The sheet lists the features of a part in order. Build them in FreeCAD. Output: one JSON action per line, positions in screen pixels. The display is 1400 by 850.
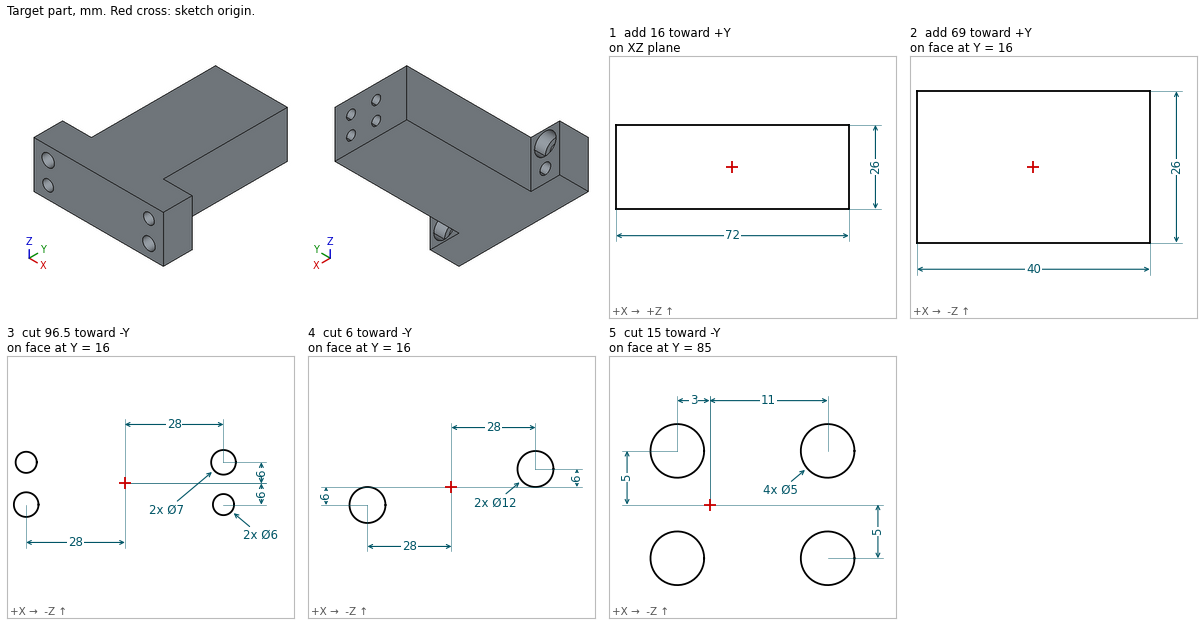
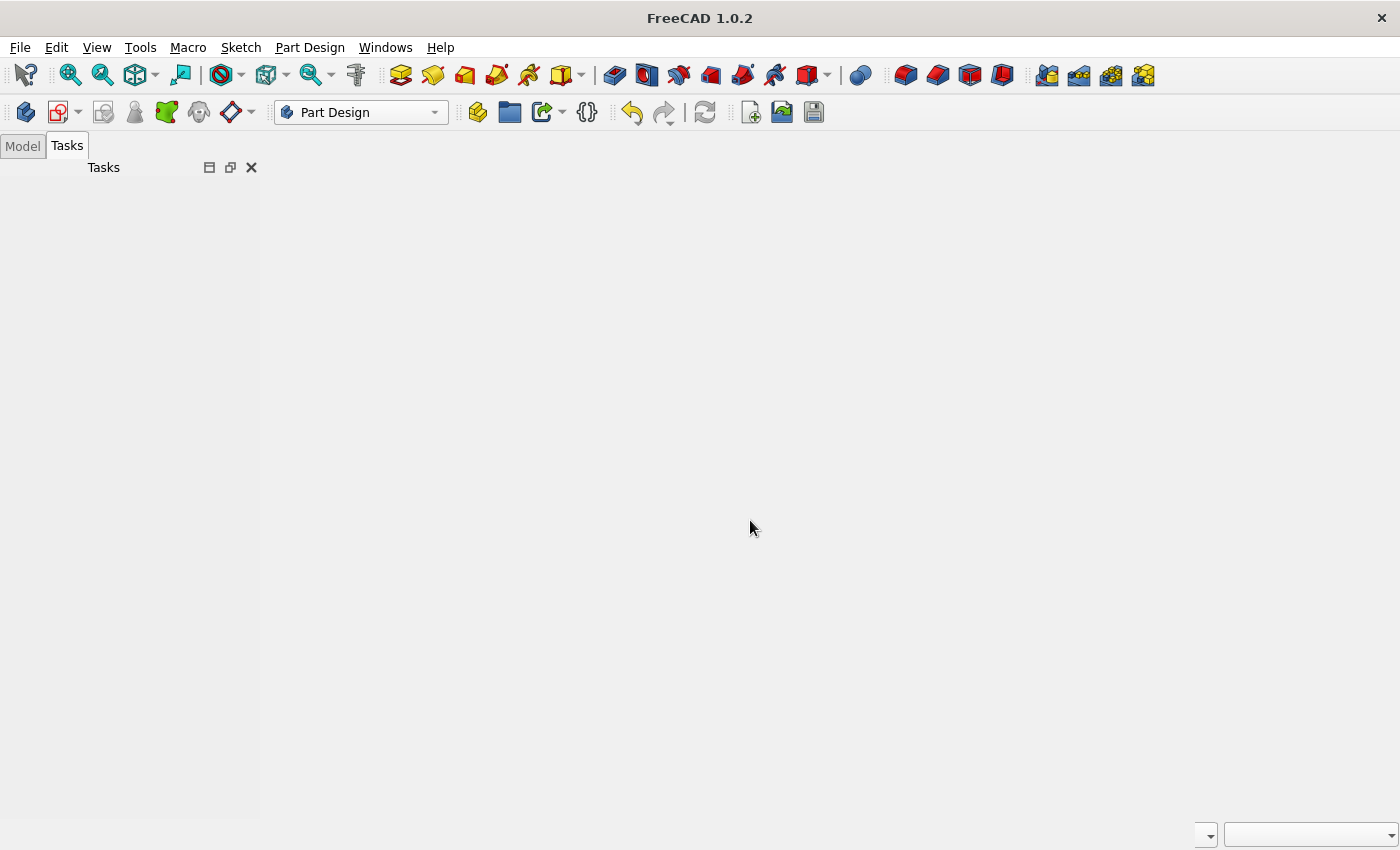
{"action": "left_click", "coordinate": [750, 112]}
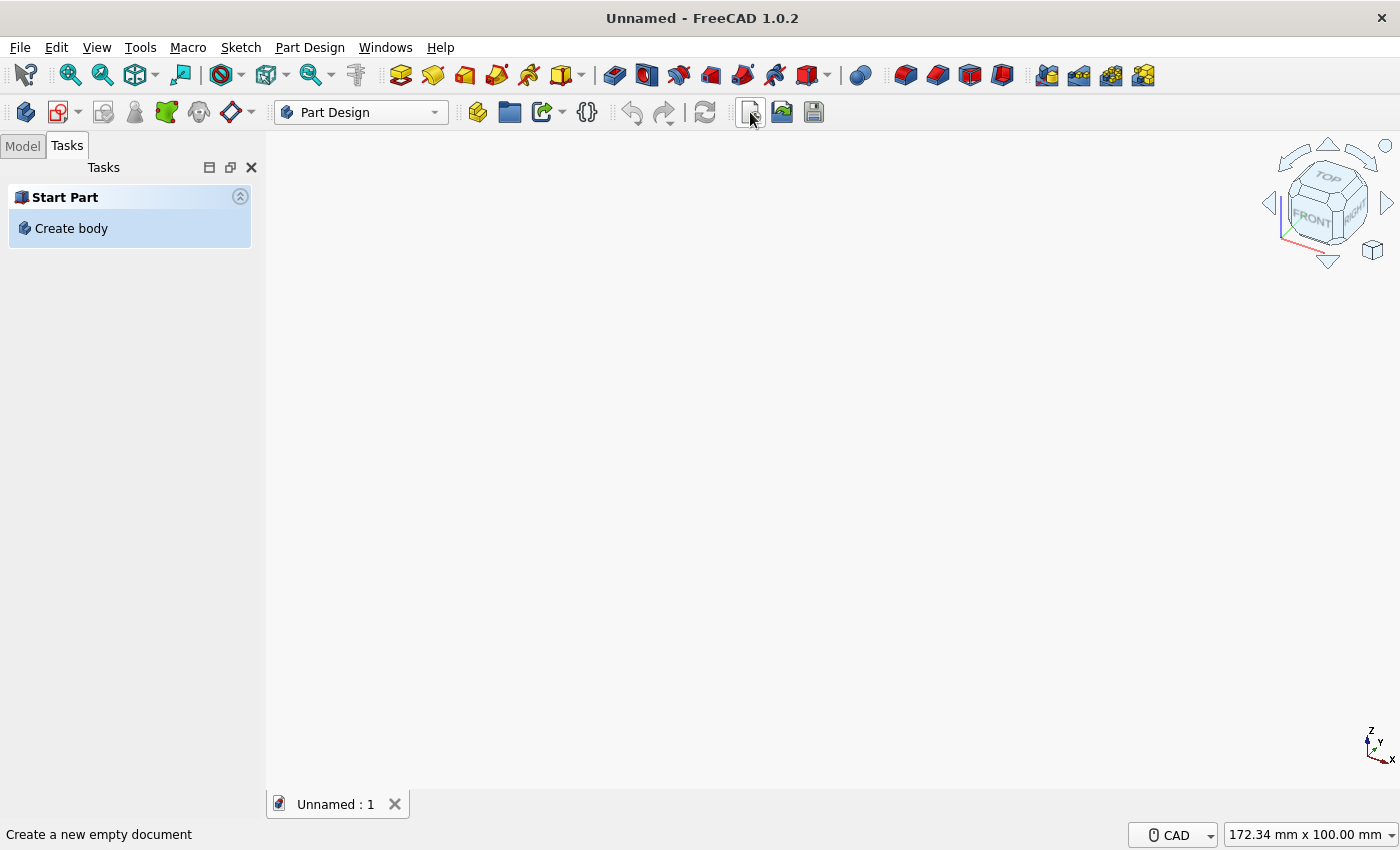
{"action": "left_click", "coordinate": [58, 112]}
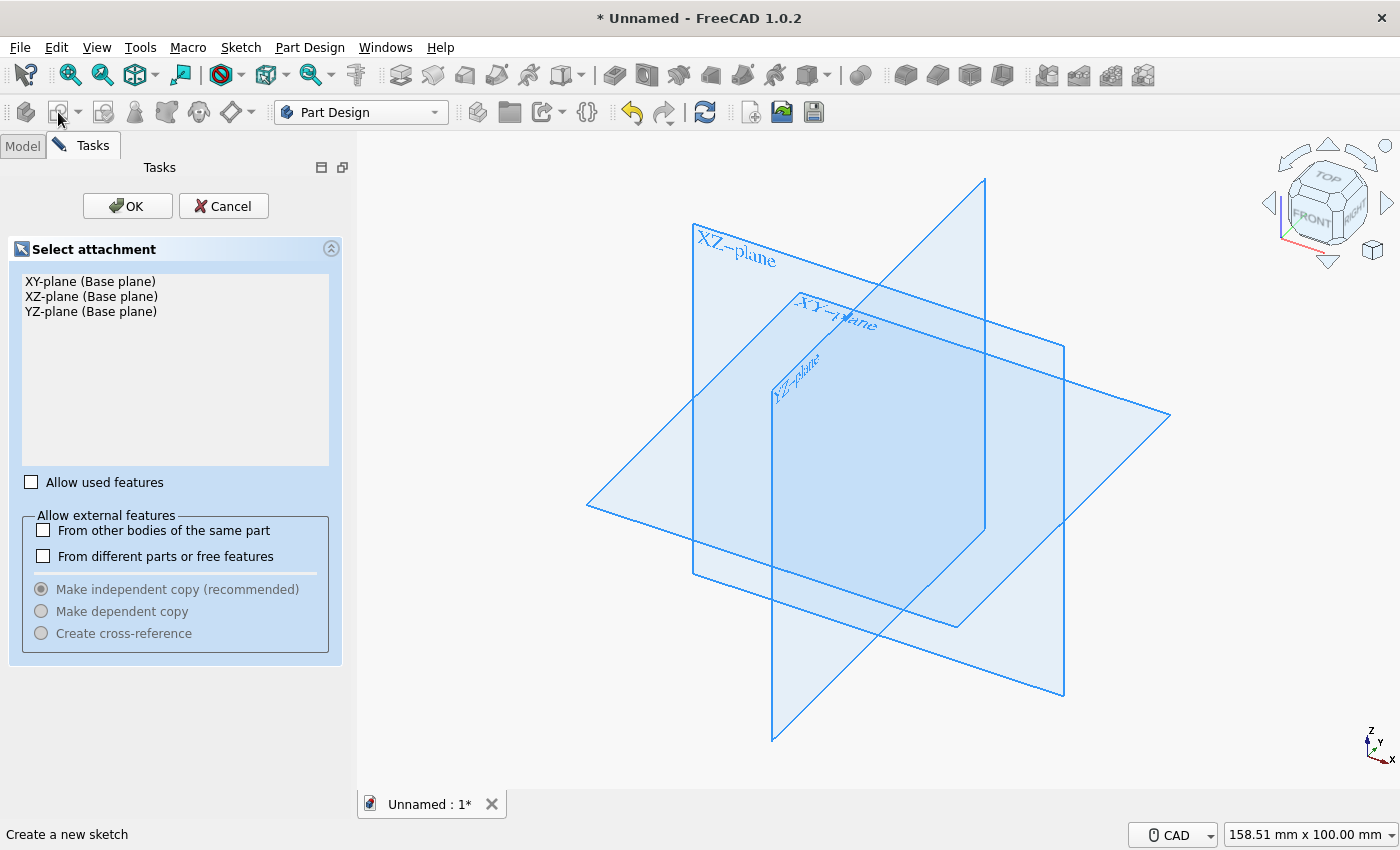
{"action": "left_click", "coordinate": [82, 296]}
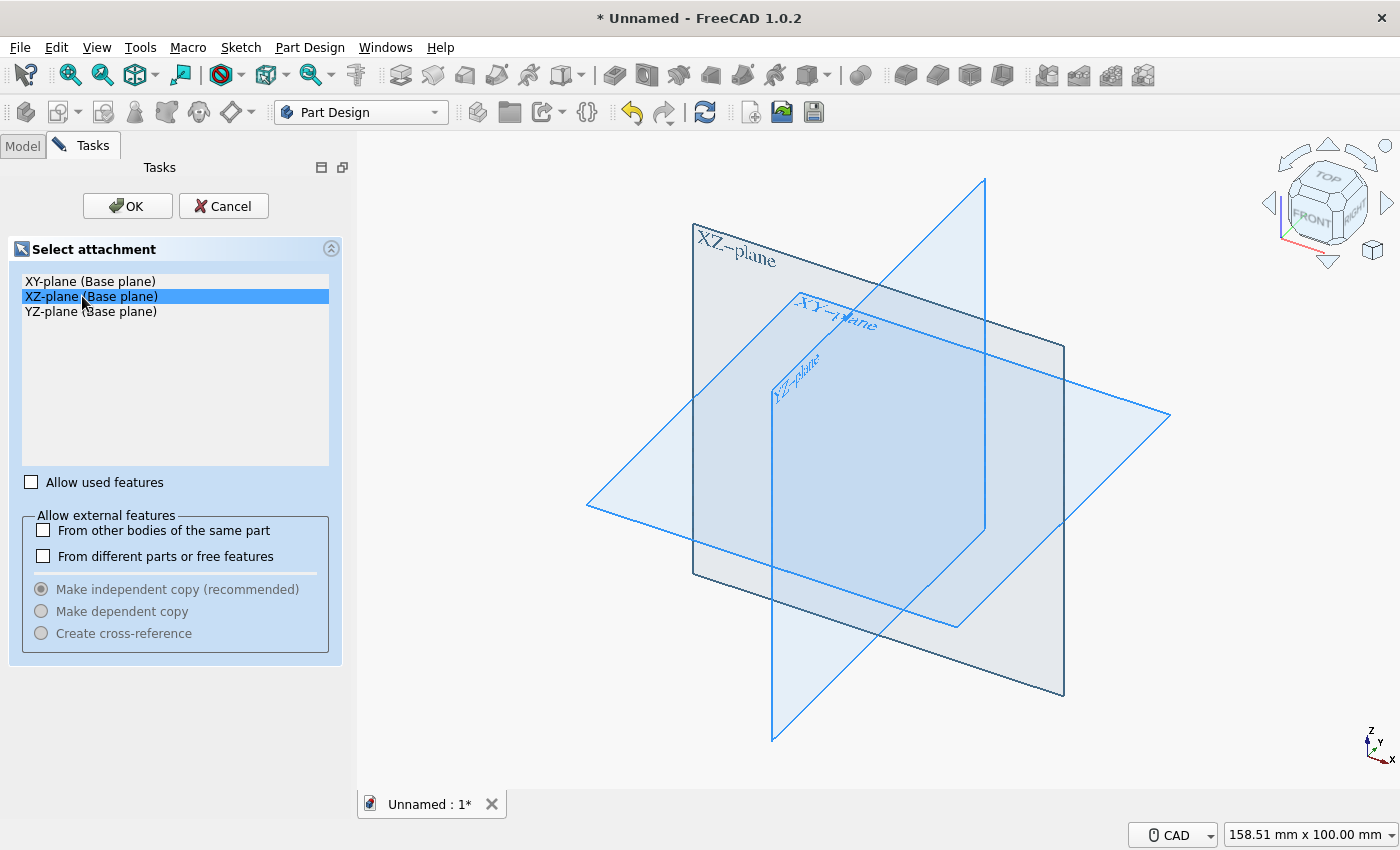
{"action": "left_click", "coordinate": [128, 206]}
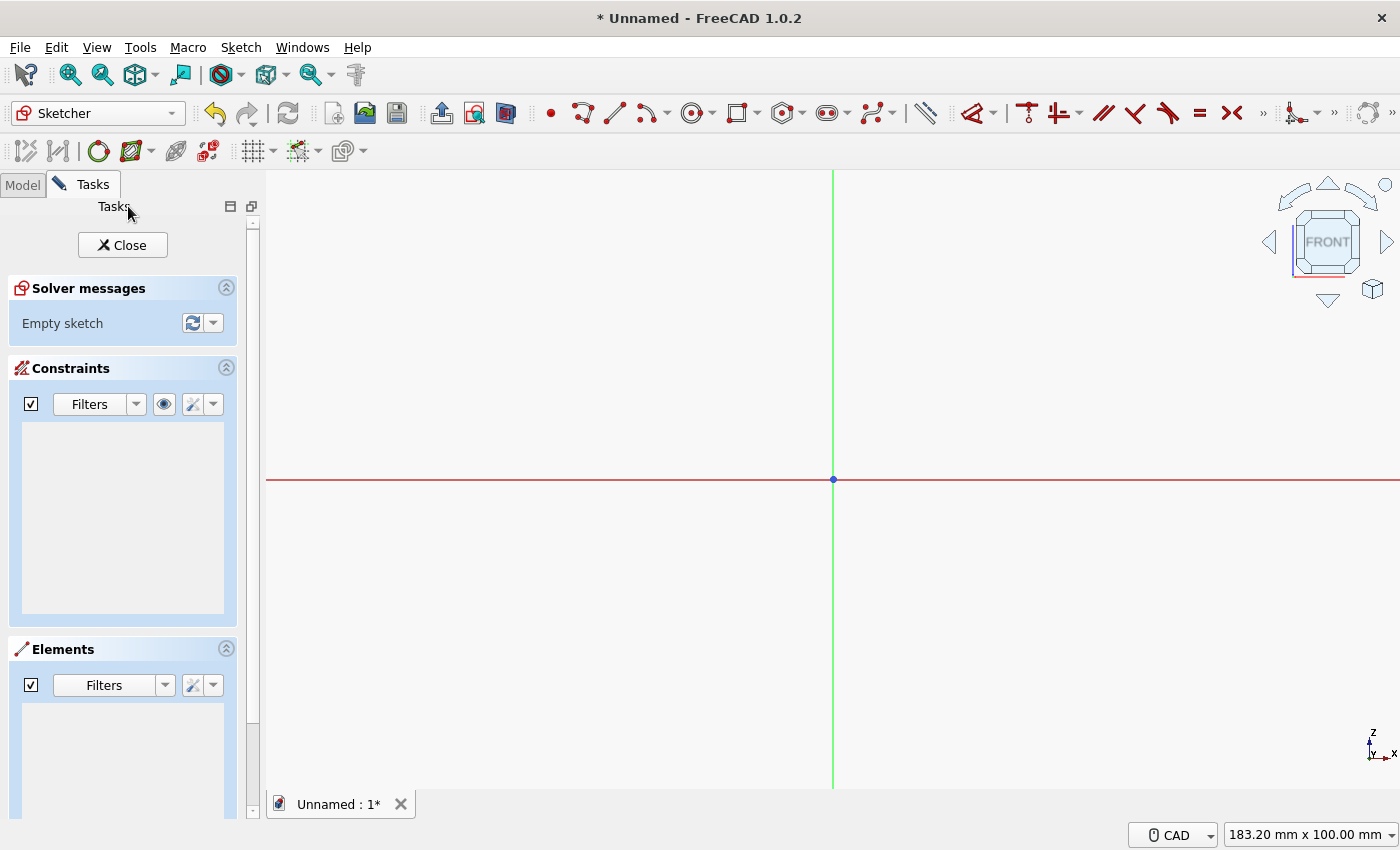
{"action": "scroll", "coordinate": [972, 480], "scroll_direction": "up", "scroll_amount": 2}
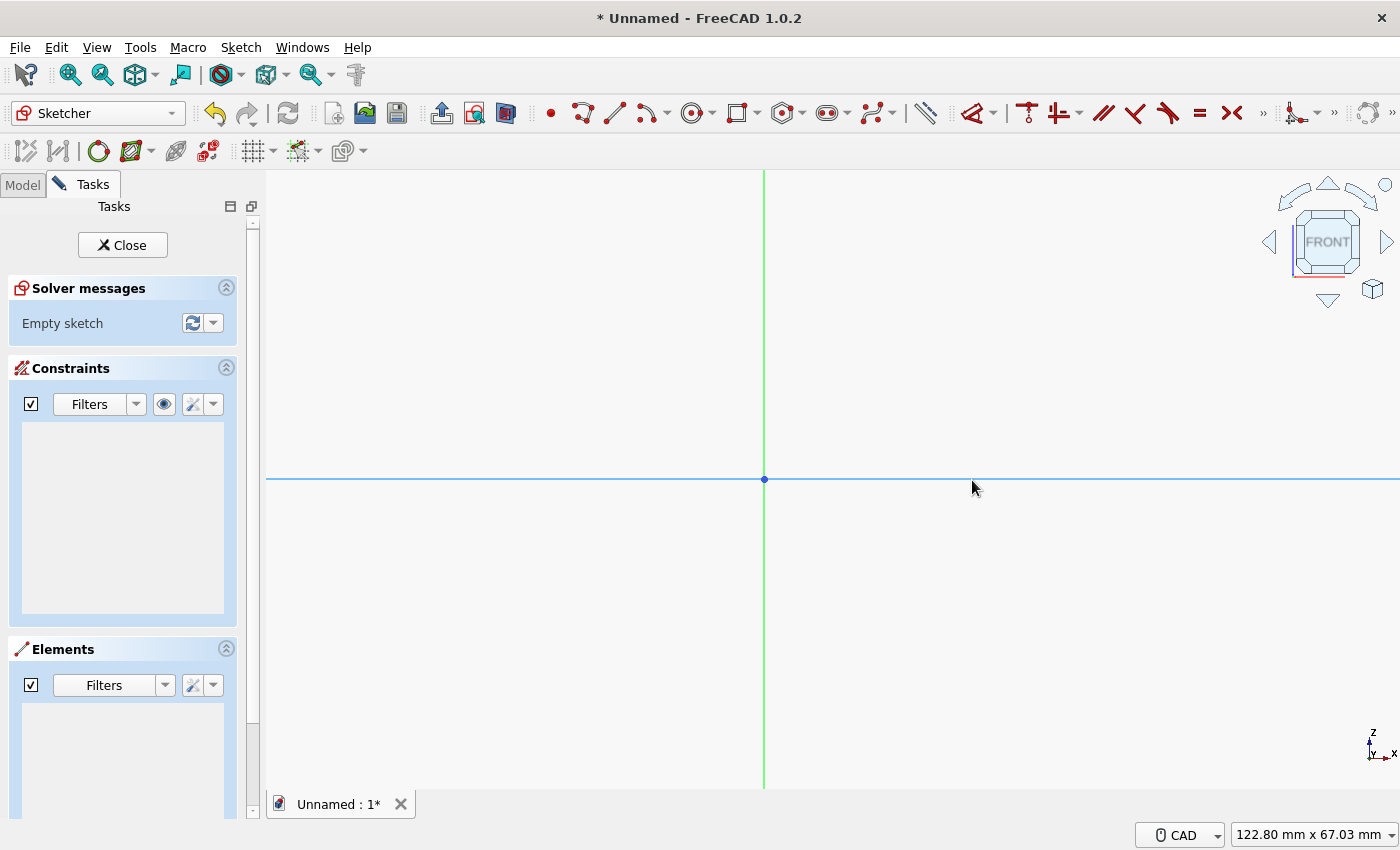
{"action": "key", "text": "g v"}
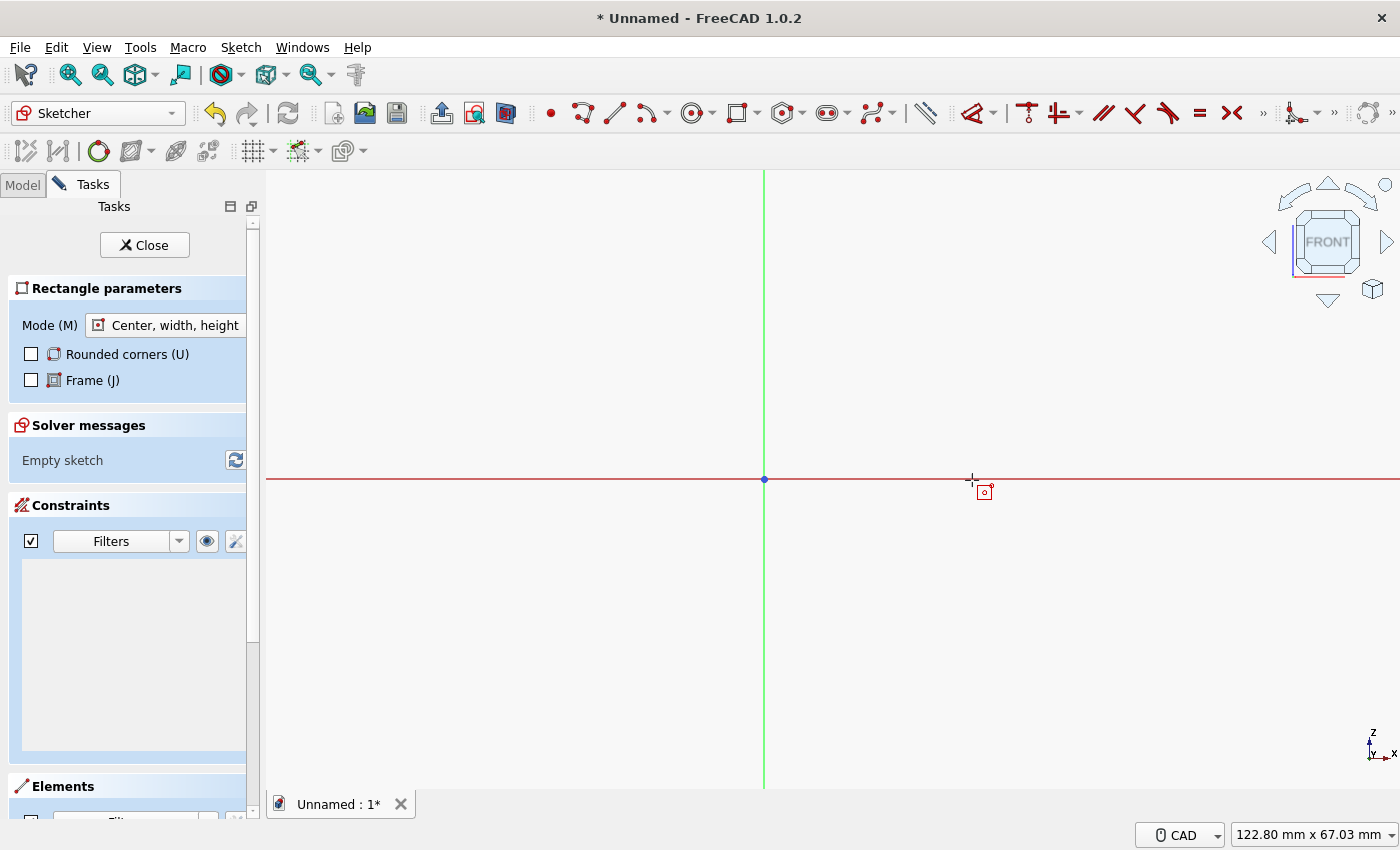
{"action": "left_click", "coordinate": [764, 479]}
{"action": "mouse_move", "coordinate": [1097, 359]}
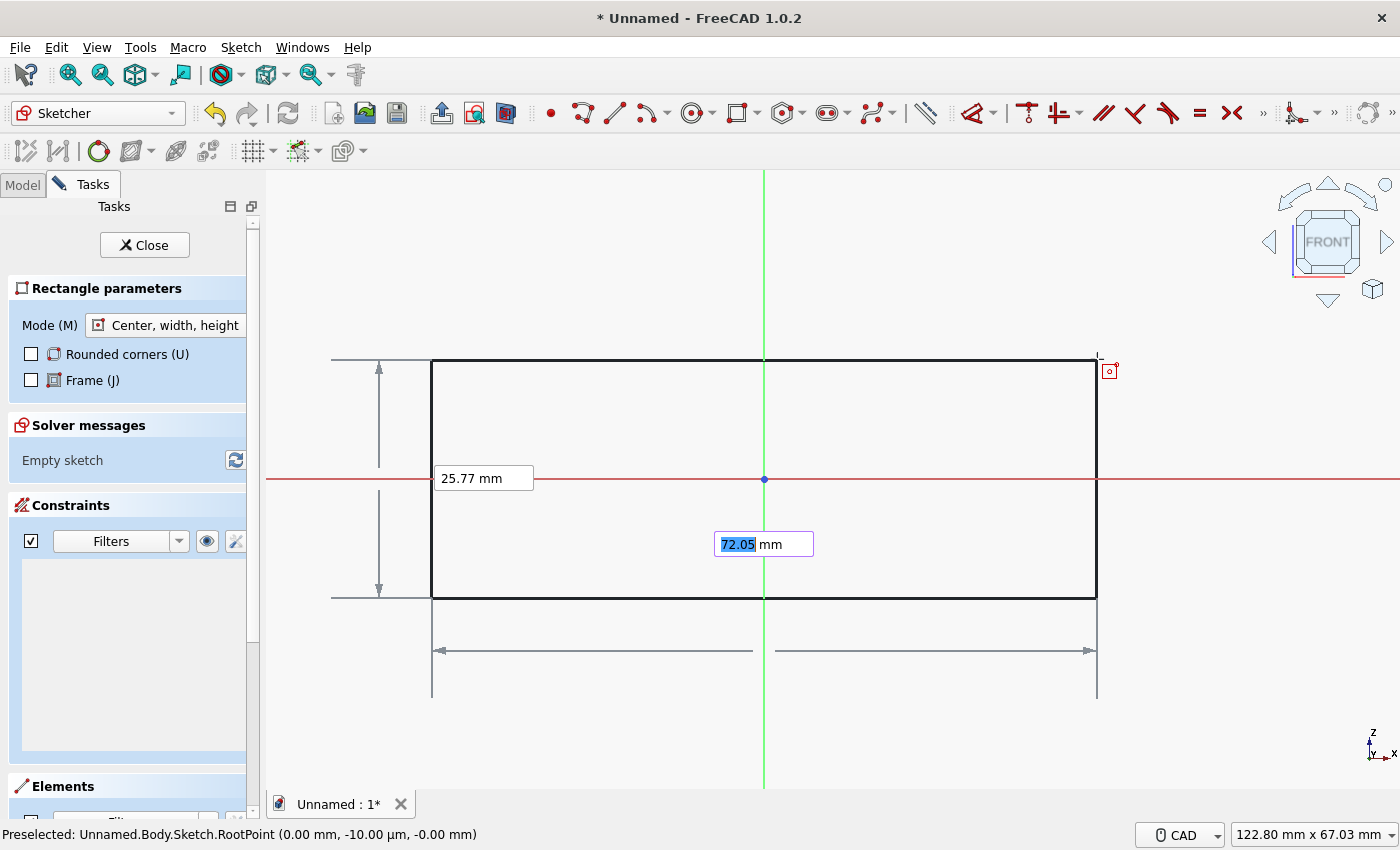
{"action": "type", "text": "72"}
{"action": "key", "text": "Tab"}
{"action": "type", "text": "26"}
{"action": "key", "text": "Return"}
{"action": "key", "text": "Escape"}